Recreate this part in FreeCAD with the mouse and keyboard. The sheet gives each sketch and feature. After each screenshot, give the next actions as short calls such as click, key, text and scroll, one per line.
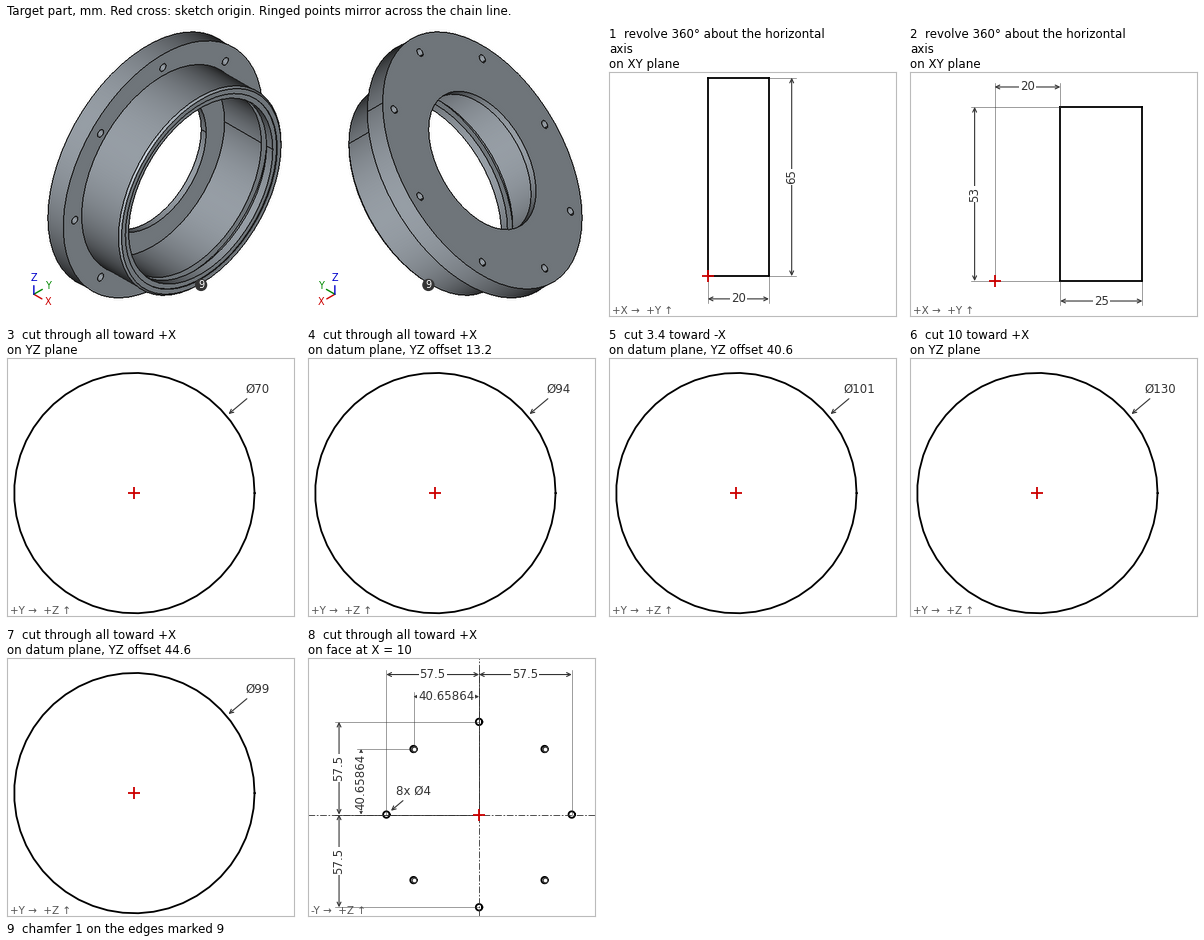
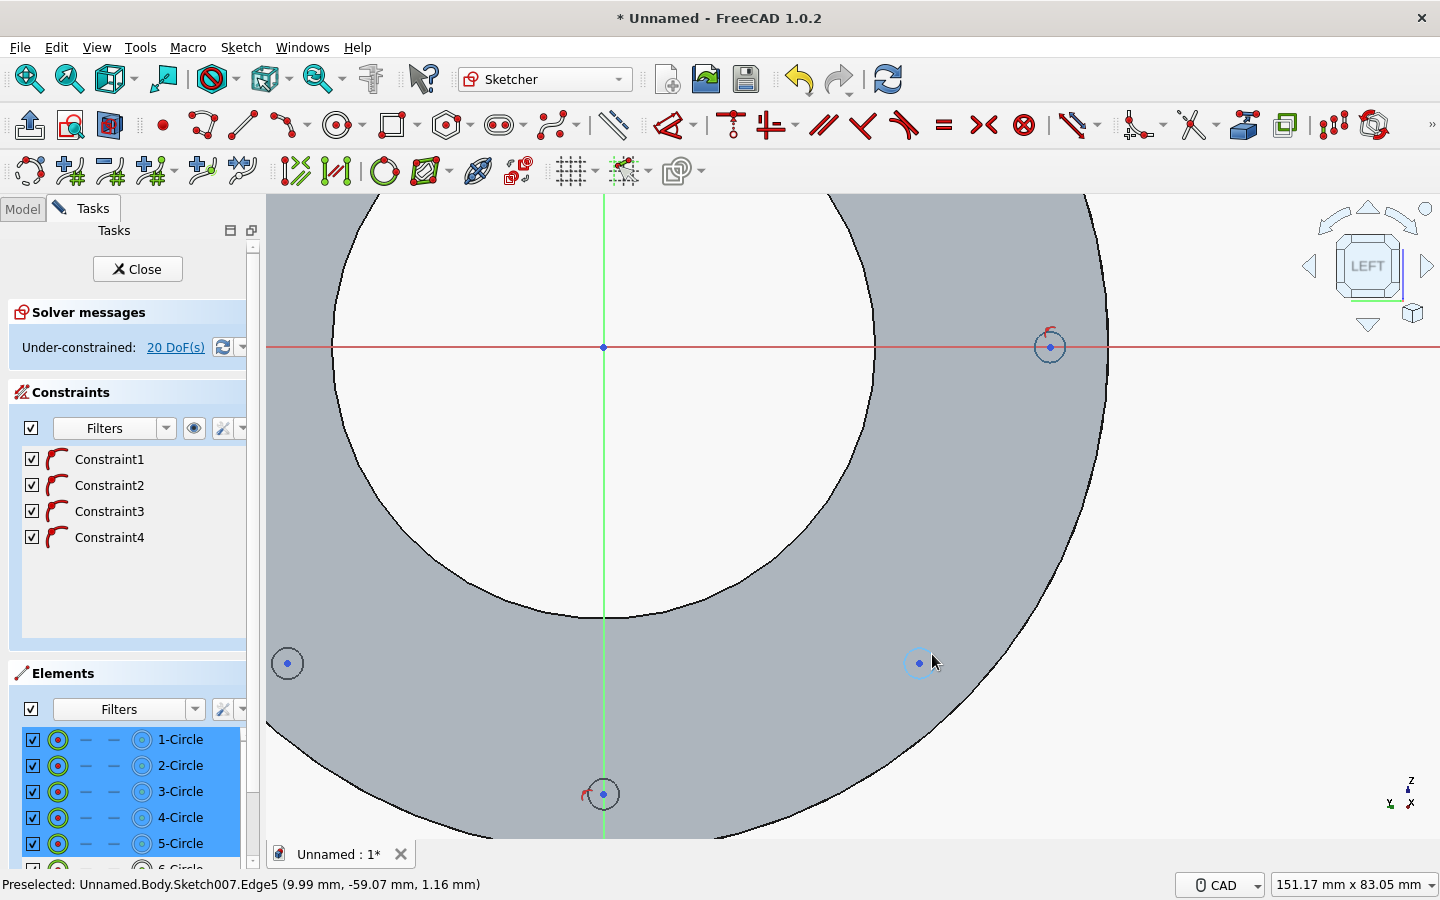
click(930, 653)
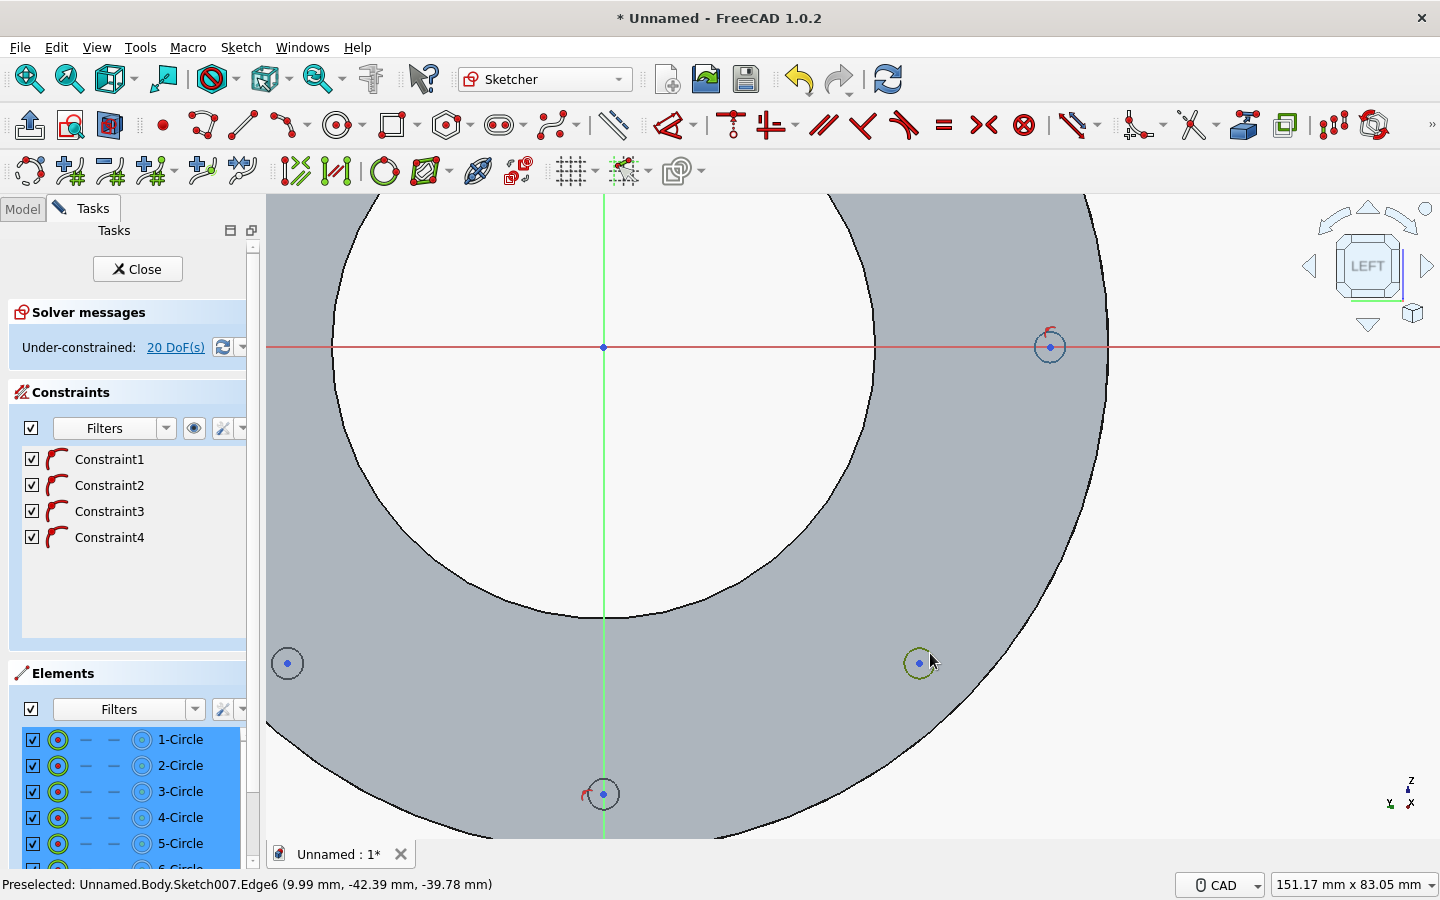
scroll(614, 783, up, 2)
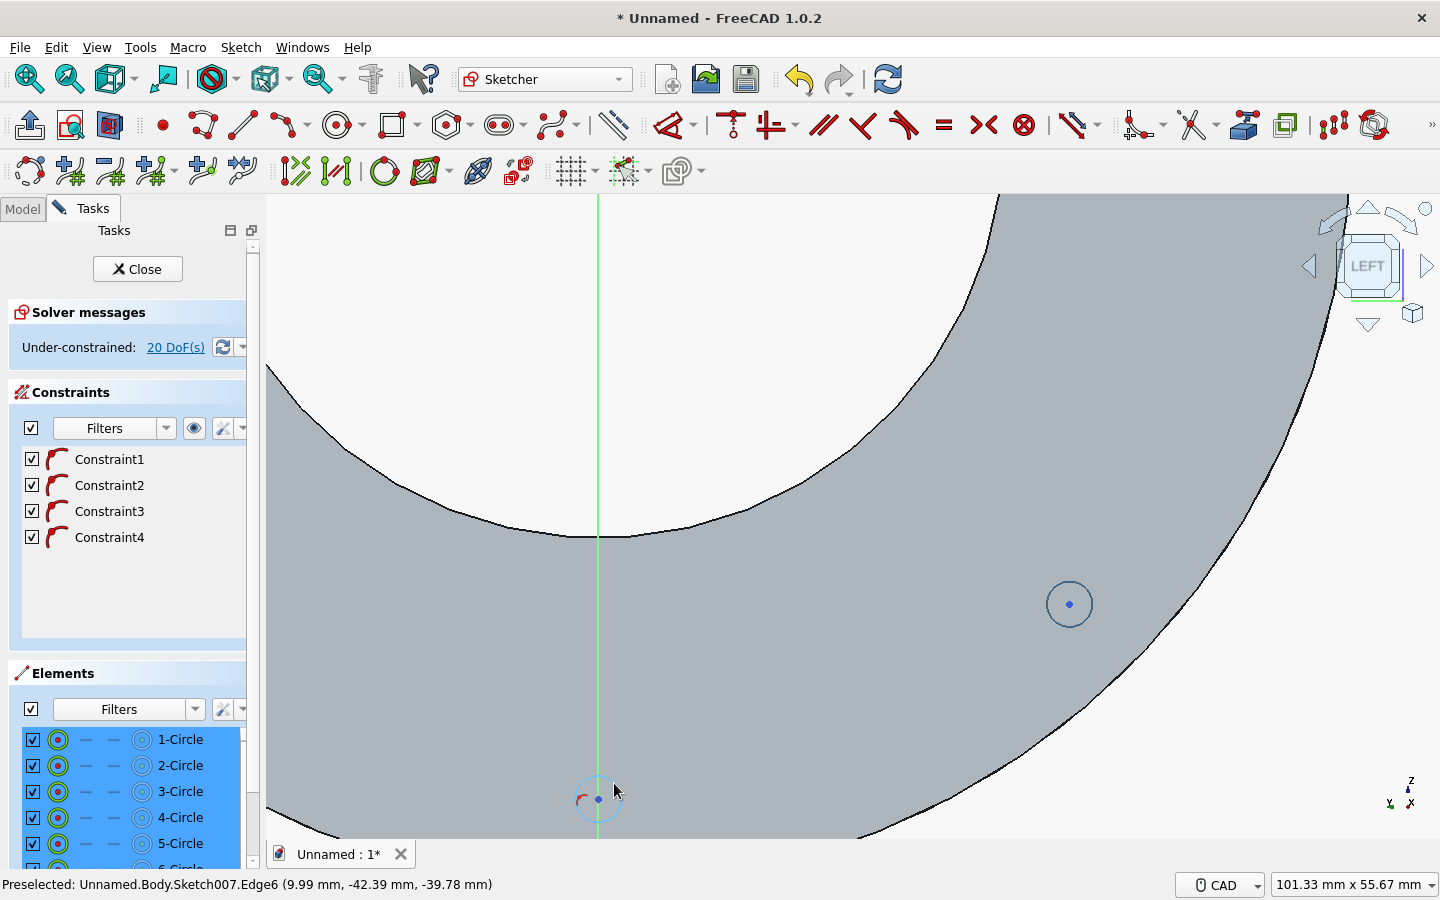
click(615, 783)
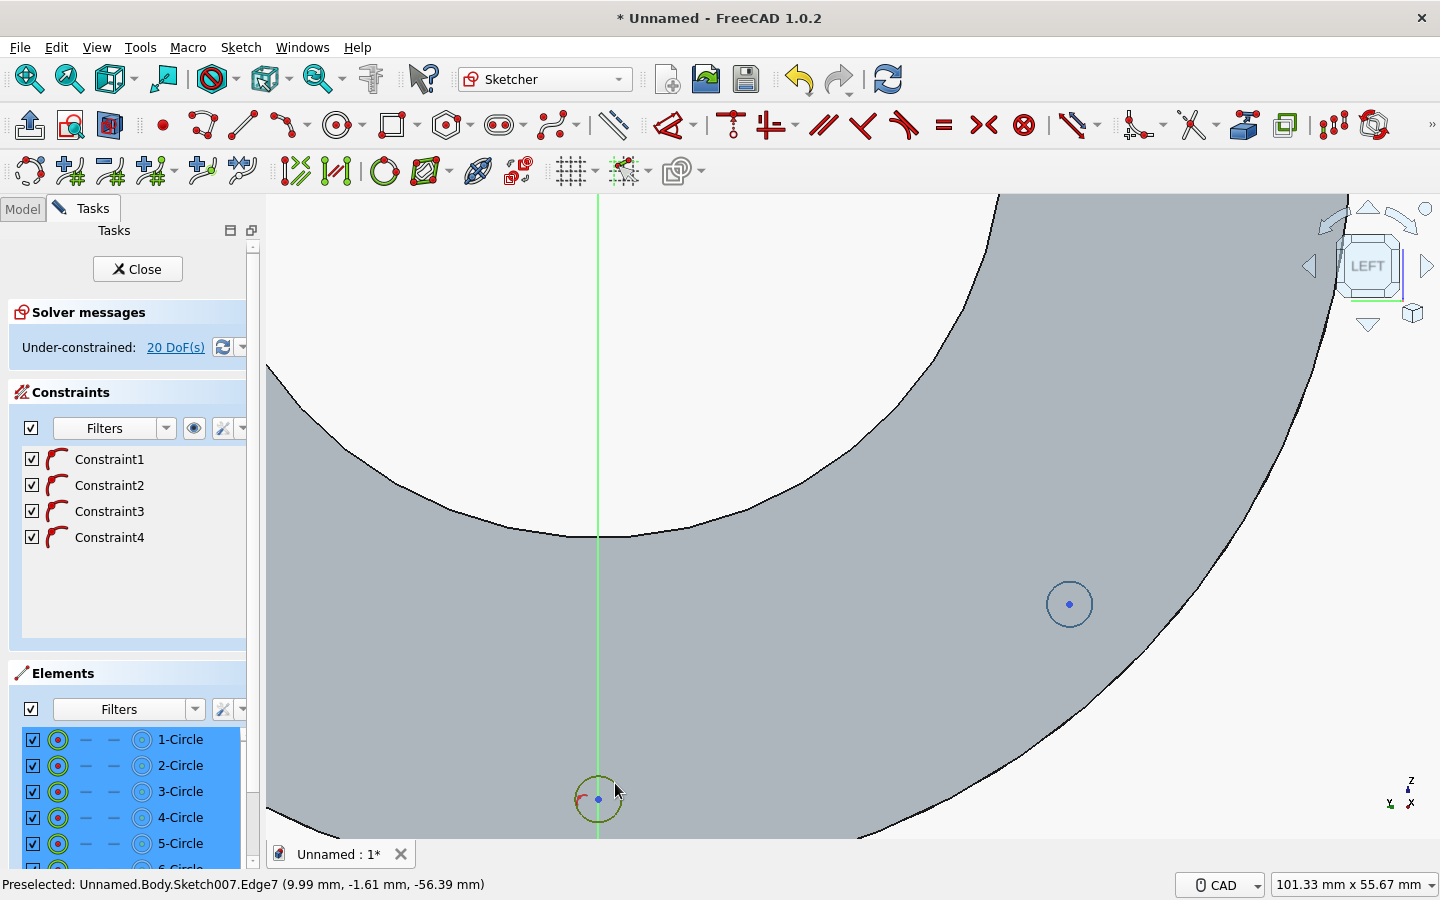
scroll(865, 682, down, 6)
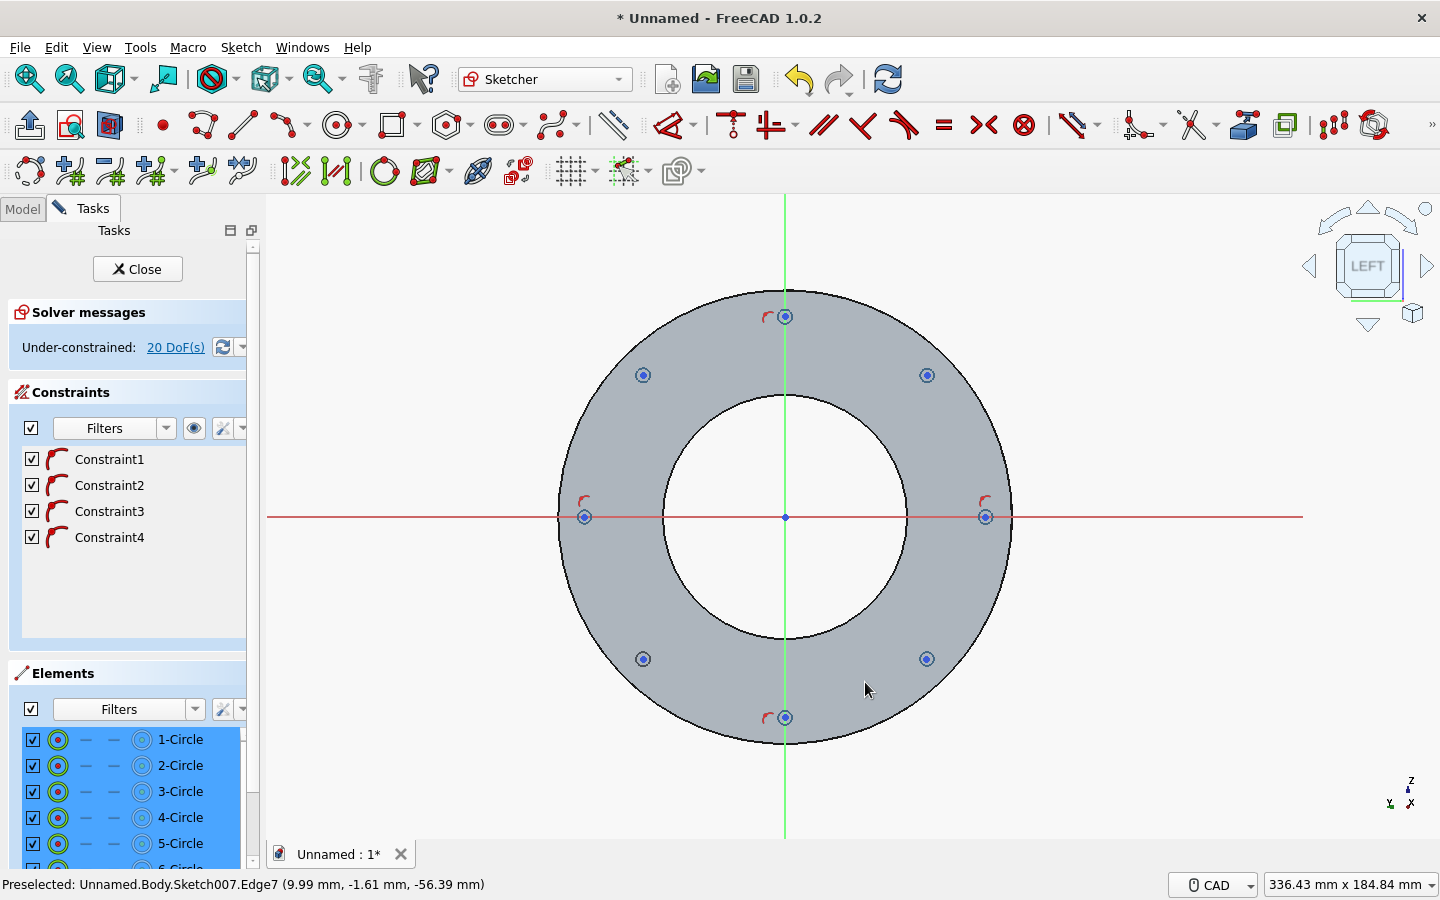
scroll(648, 654, up, 4)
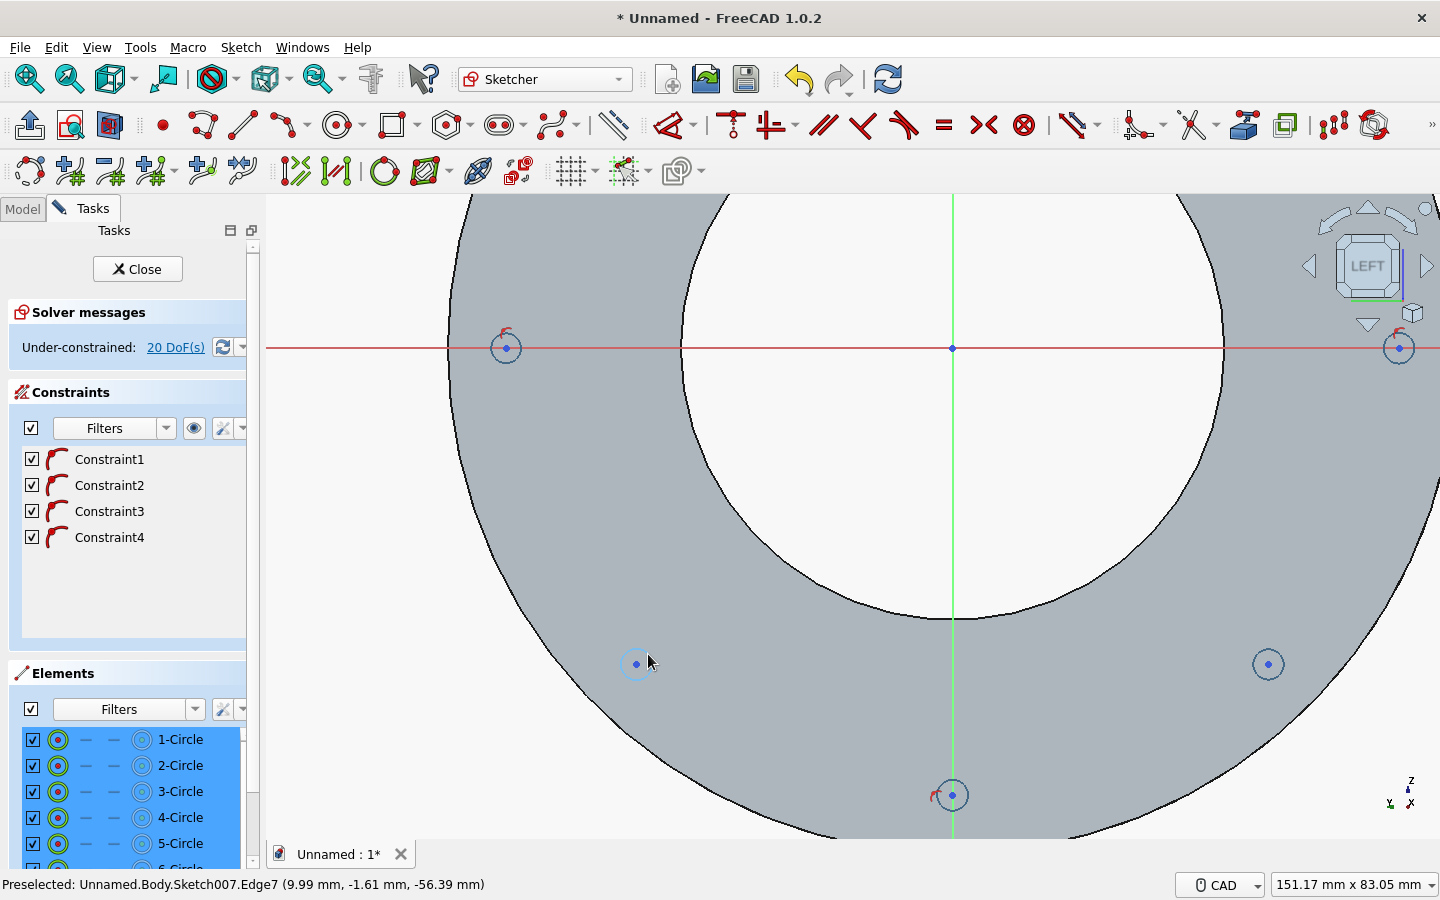
click(648, 653)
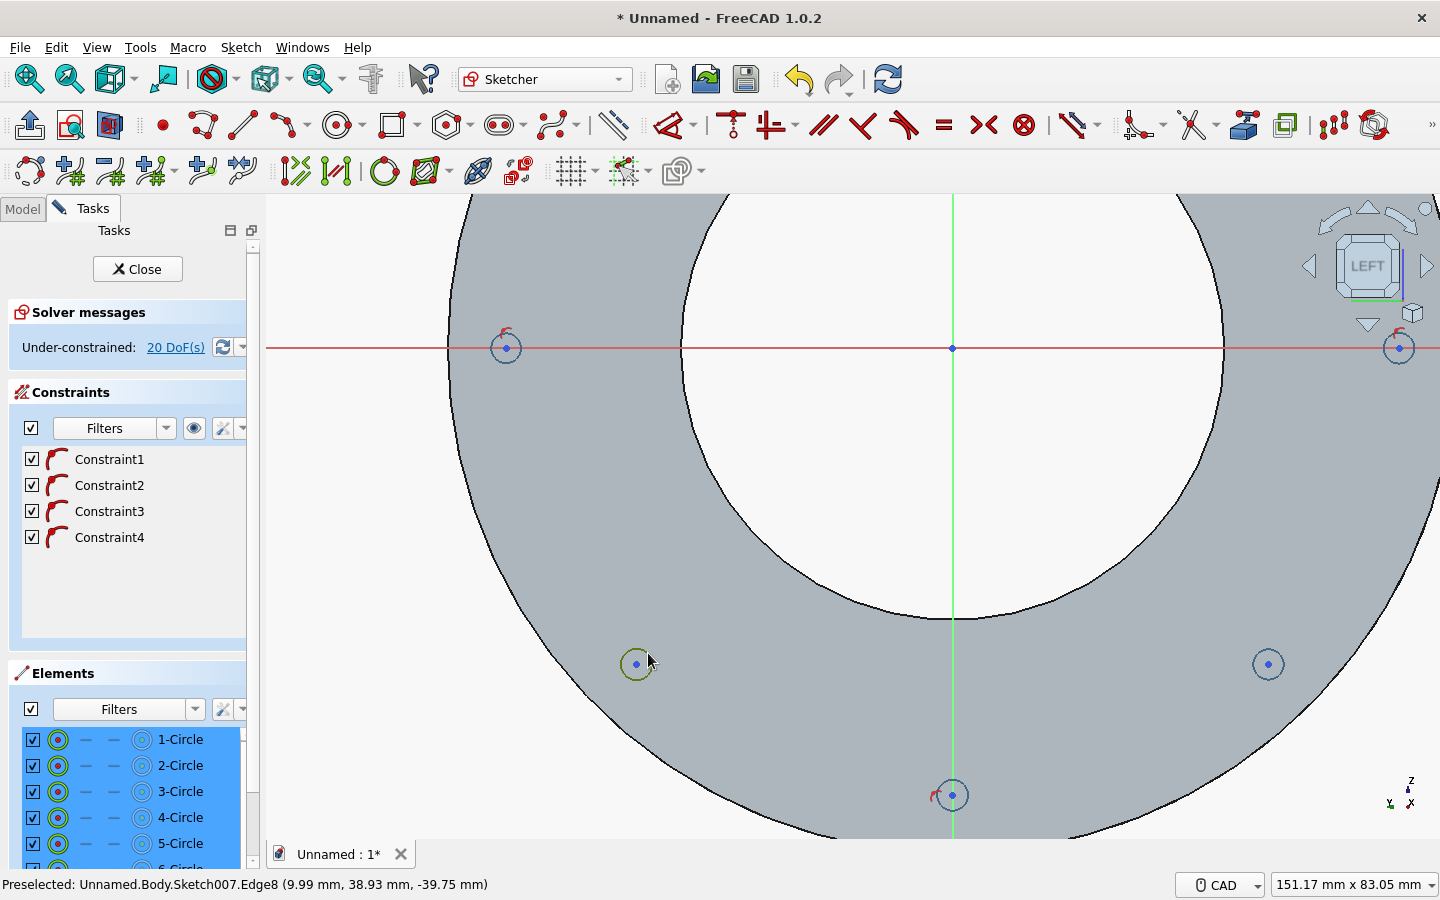
click(944, 126)